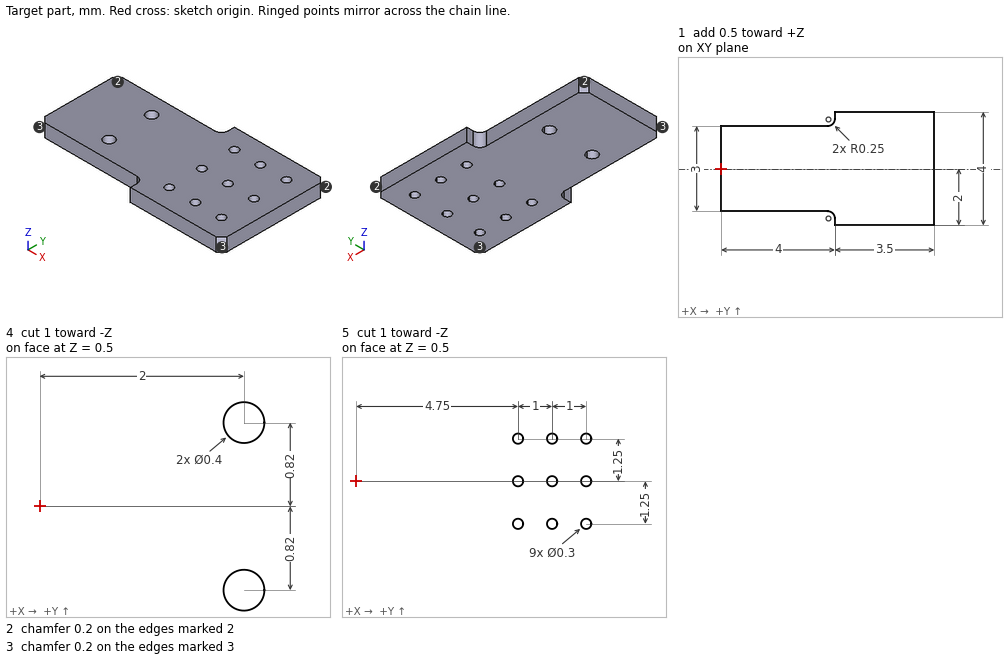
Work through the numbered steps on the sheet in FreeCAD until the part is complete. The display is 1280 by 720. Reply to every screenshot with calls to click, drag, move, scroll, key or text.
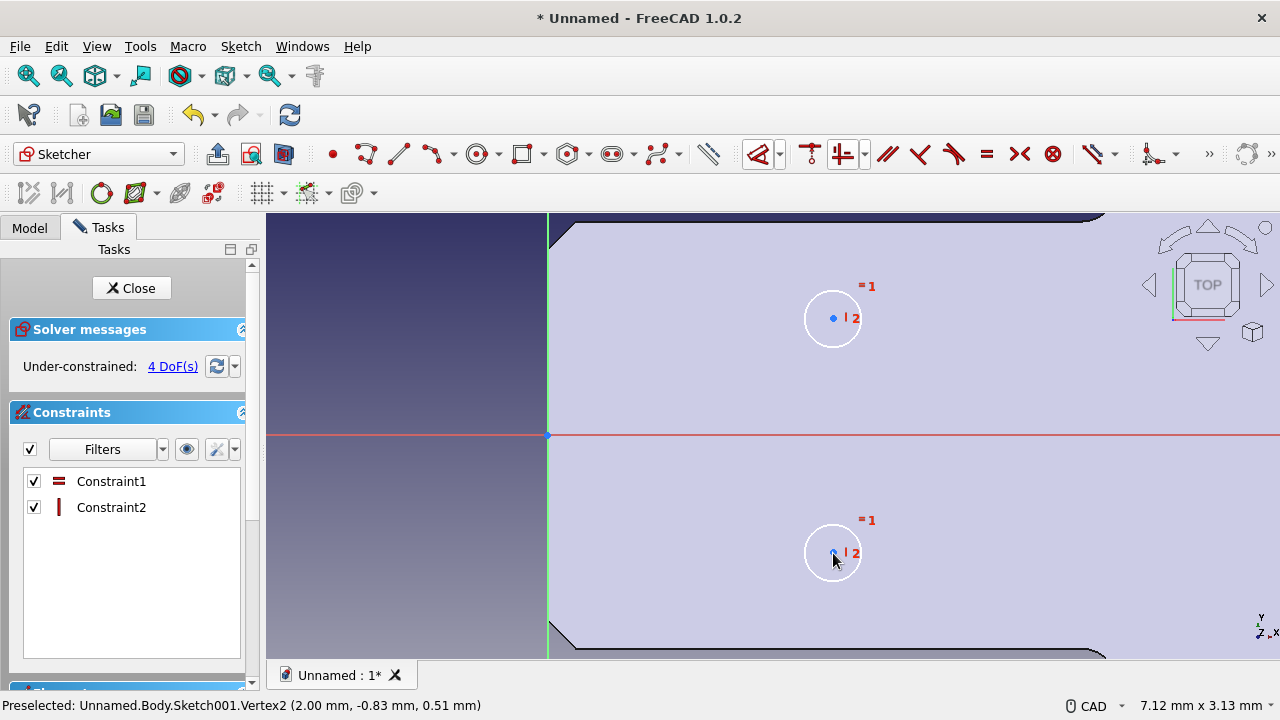
key(d)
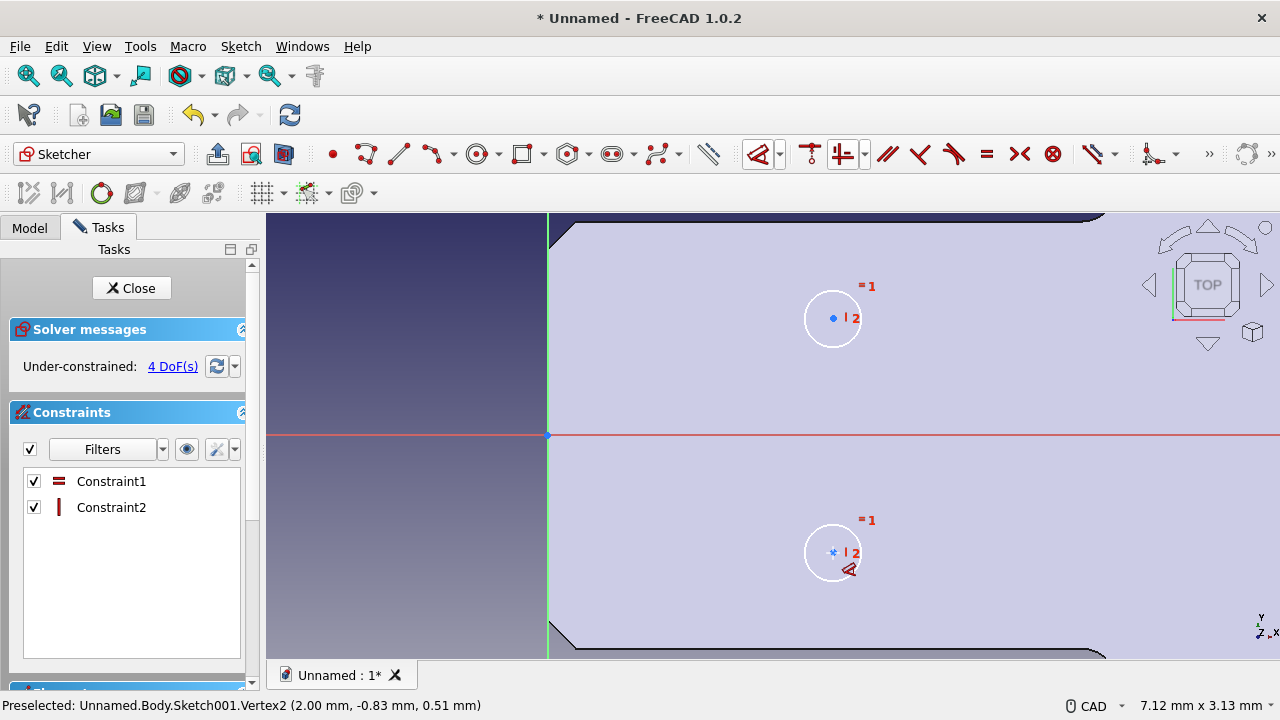
click(853, 299)
click(876, 276)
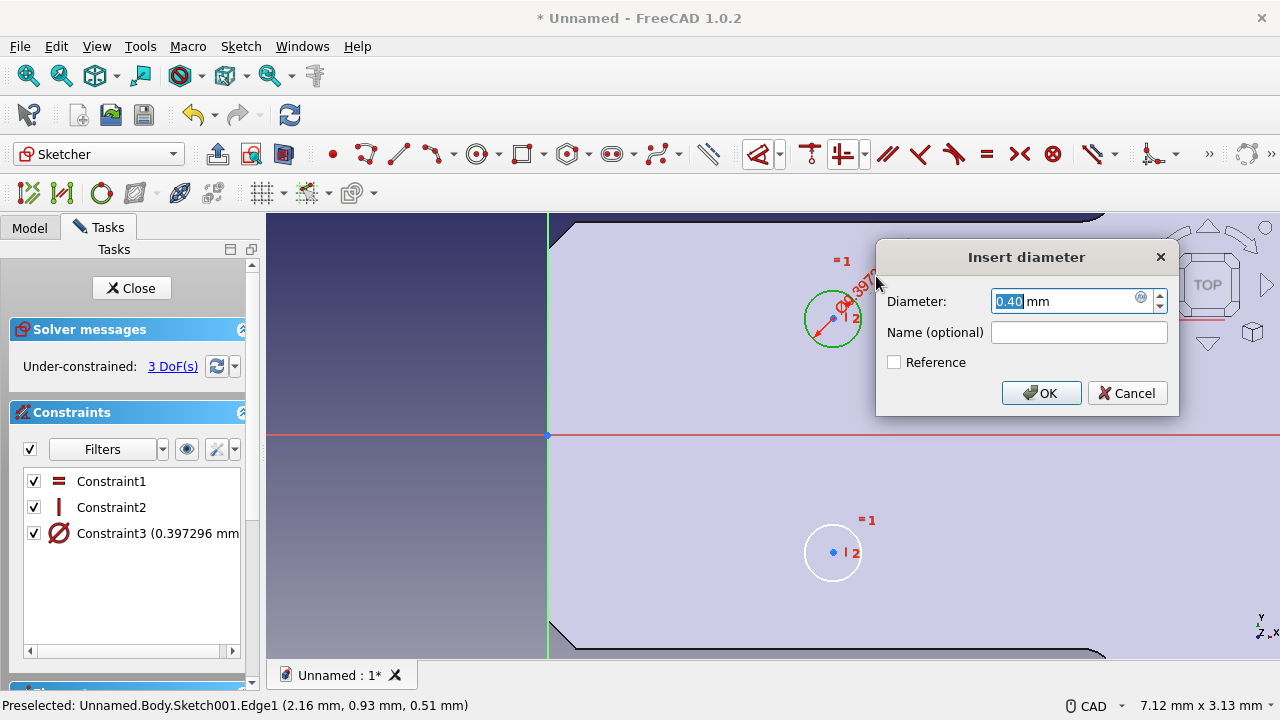
text(0.4)
key(Return)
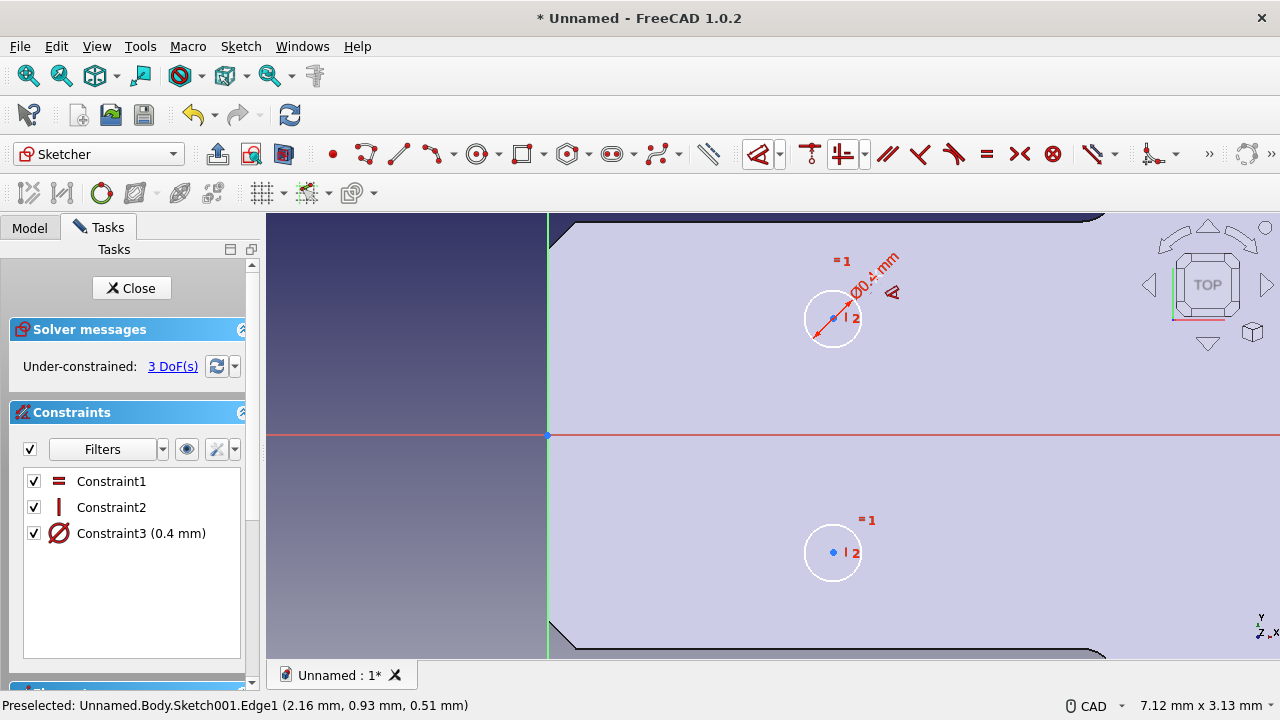
click(833, 319)
click(690, 285)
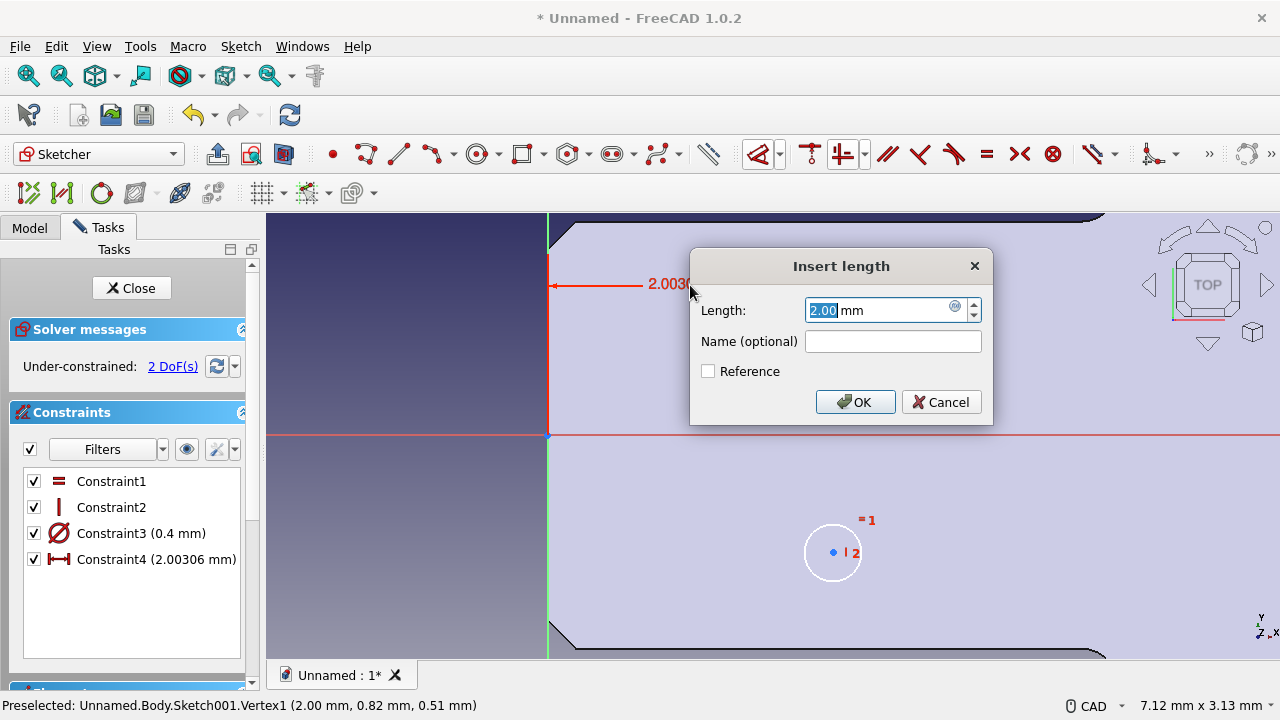
text(2)
key(Return)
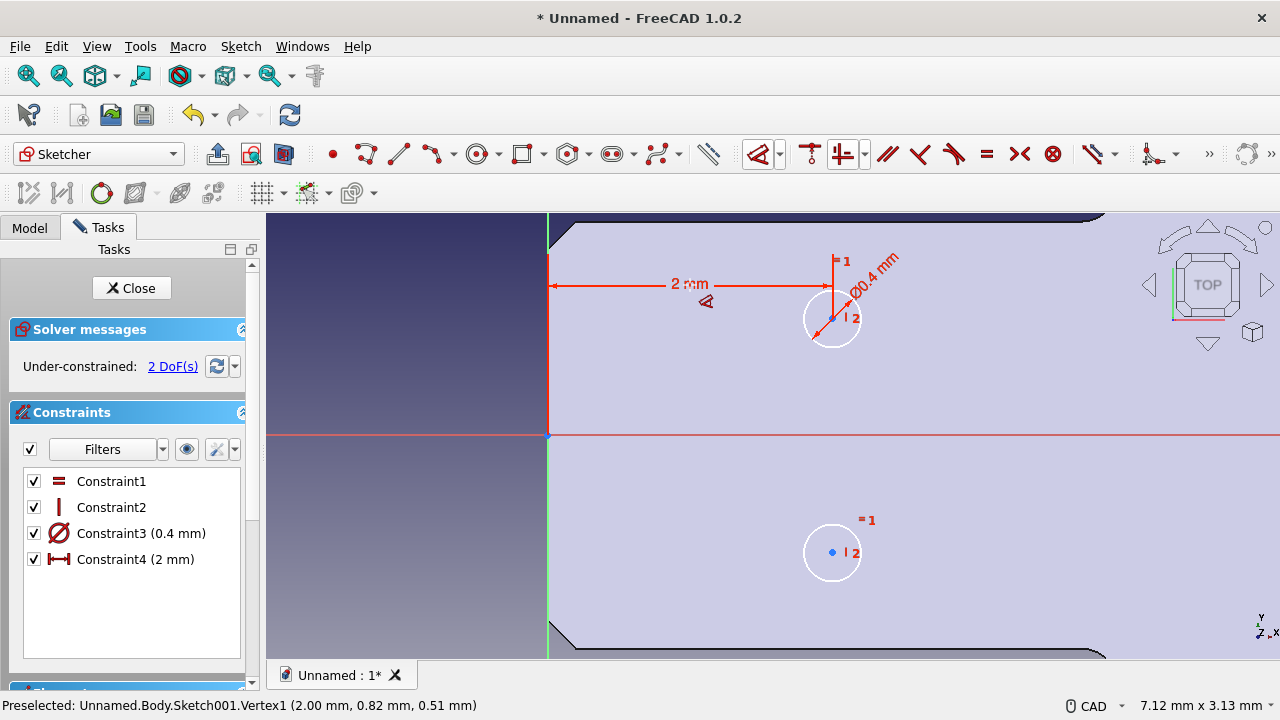
click(833, 319)
click(514, 377)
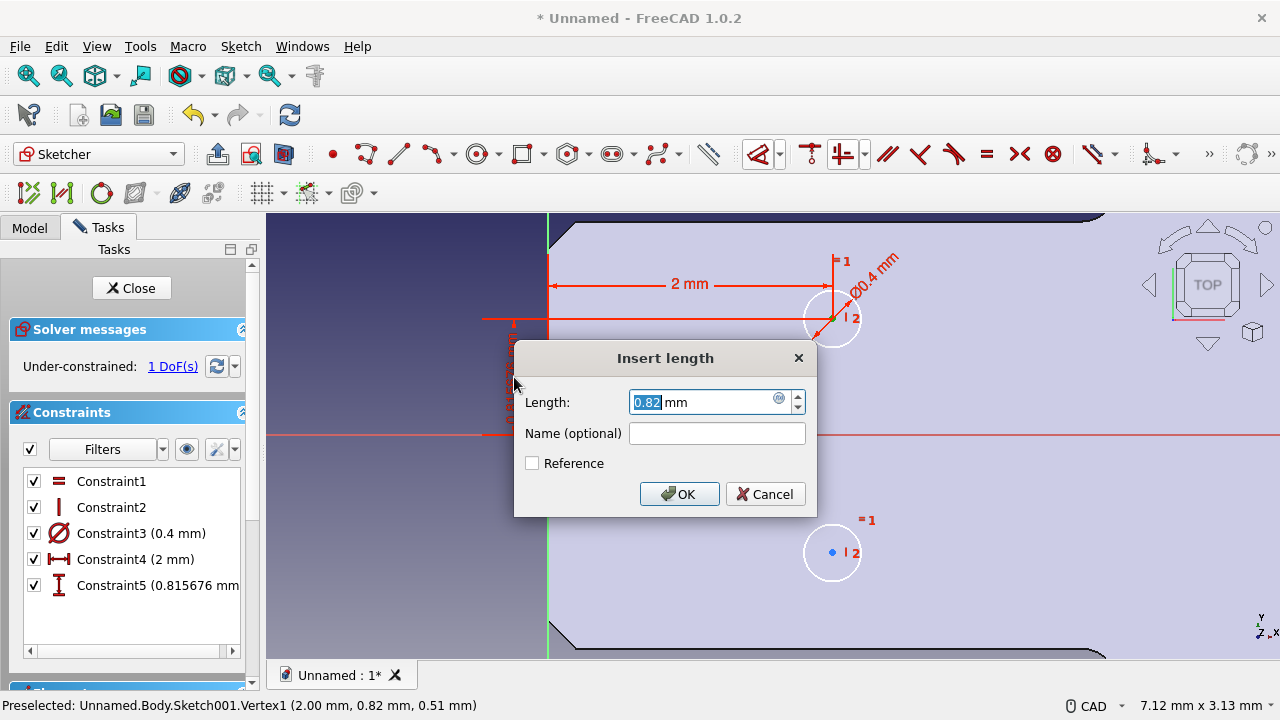
text(0.82)
key(Return)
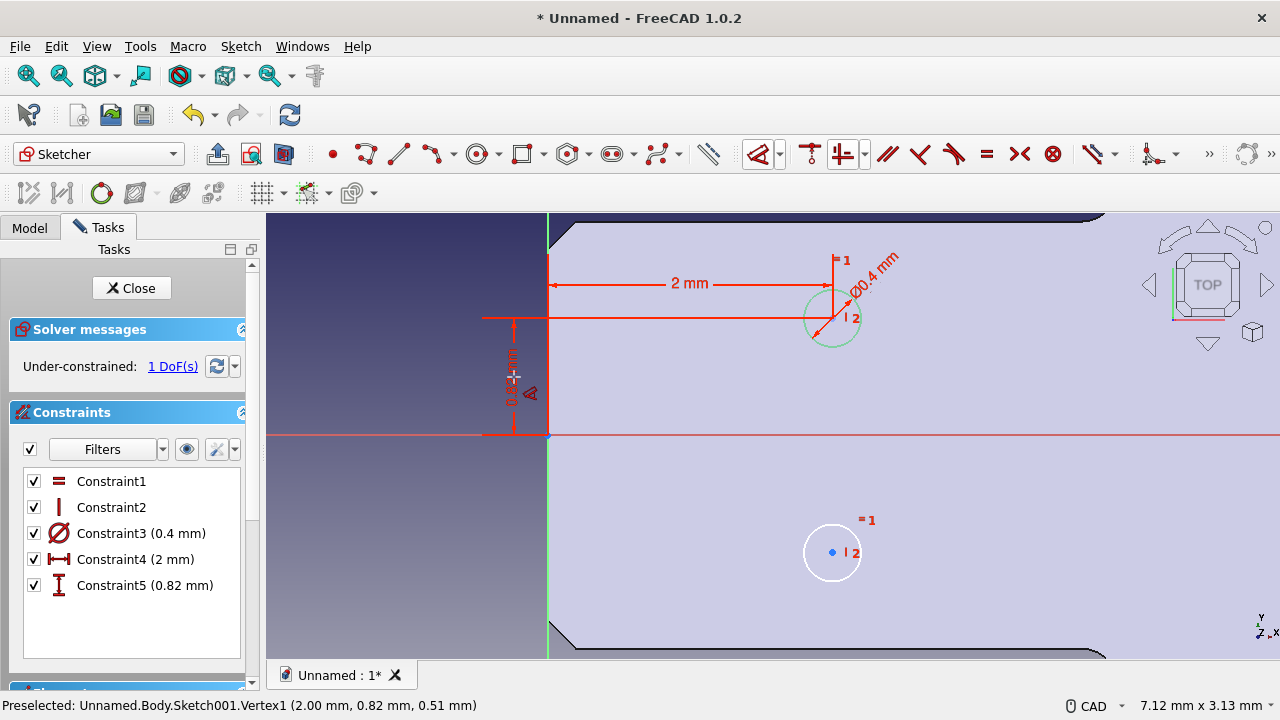
click(833, 553)
click(514, 494)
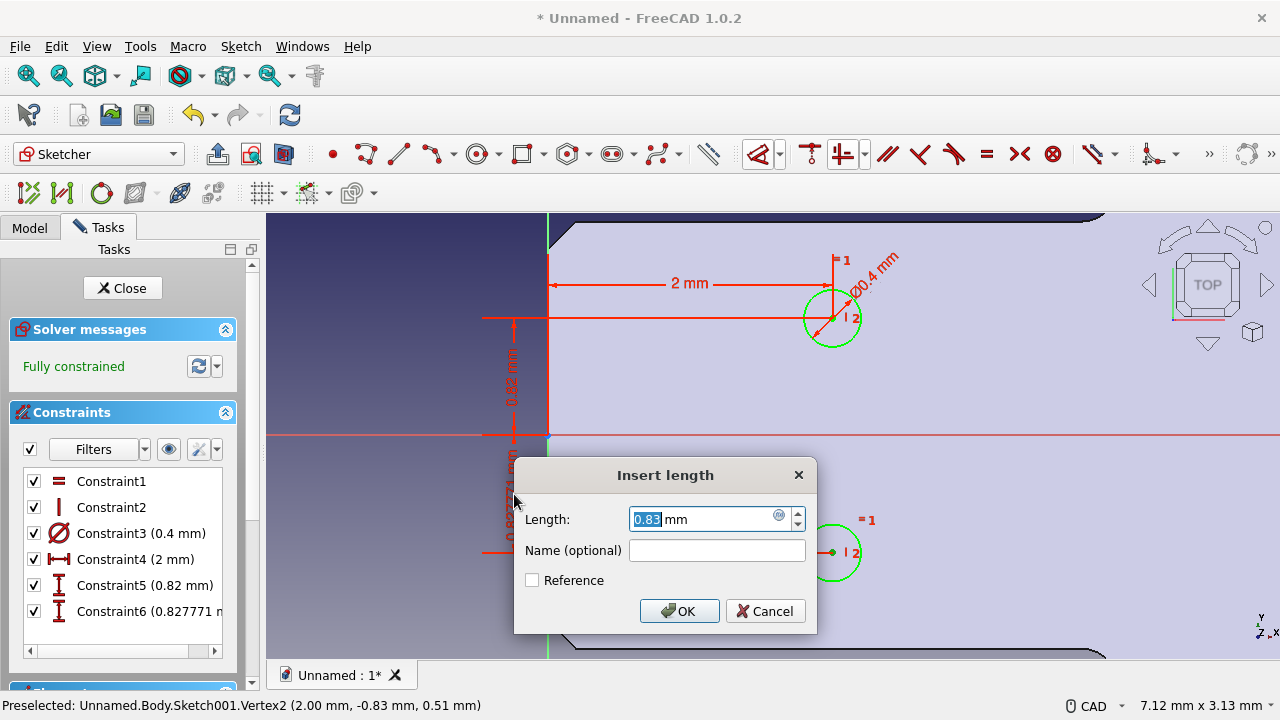
text(0.82)
key(Return)
key(Escape)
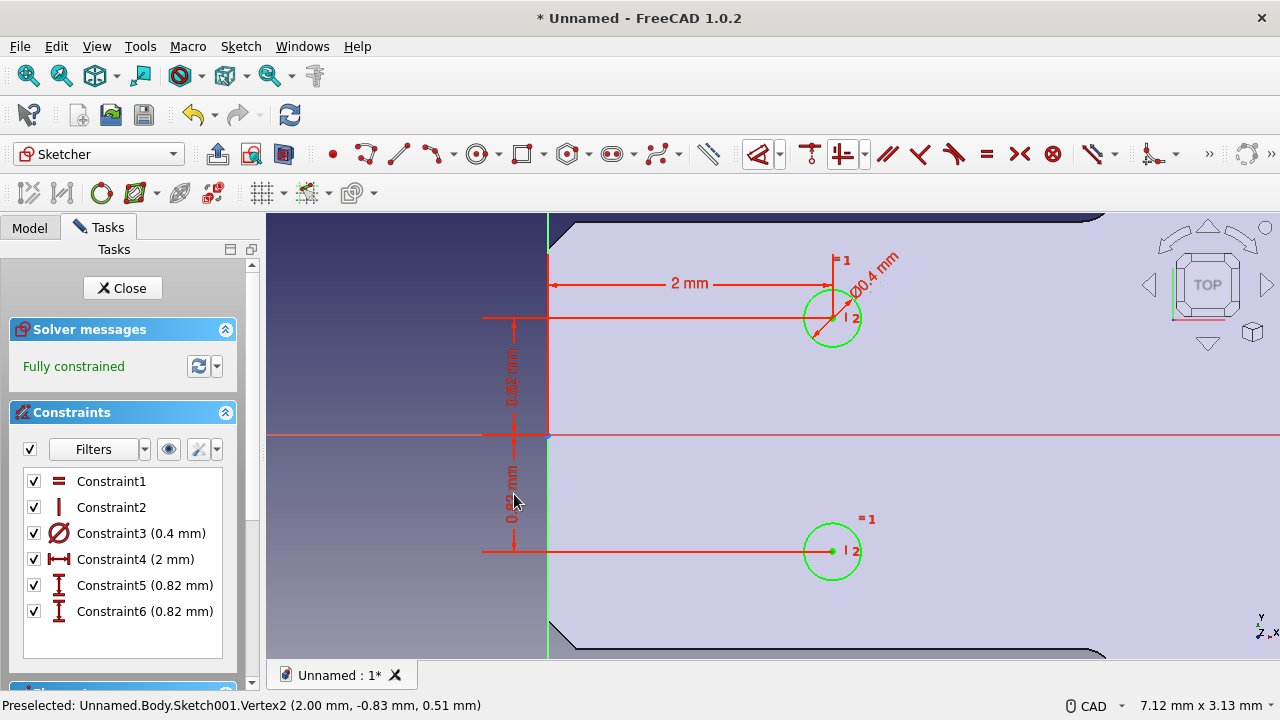
click(123, 288)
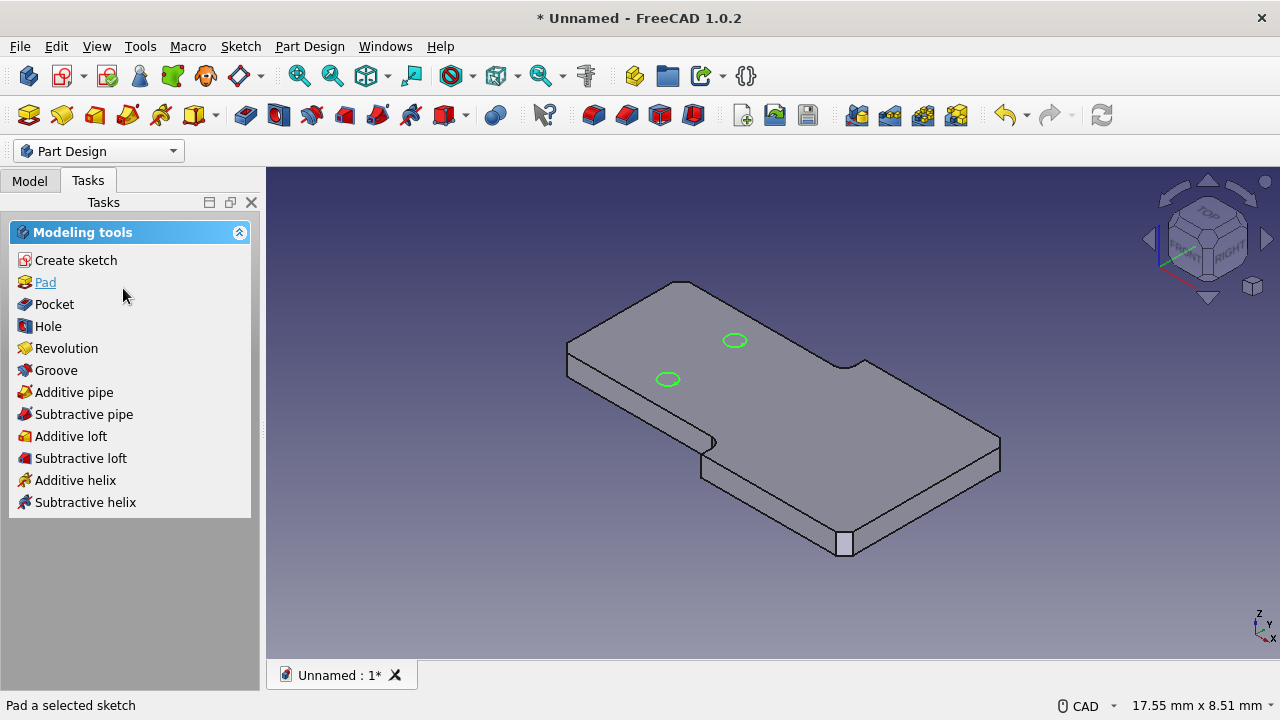
click(246, 116)